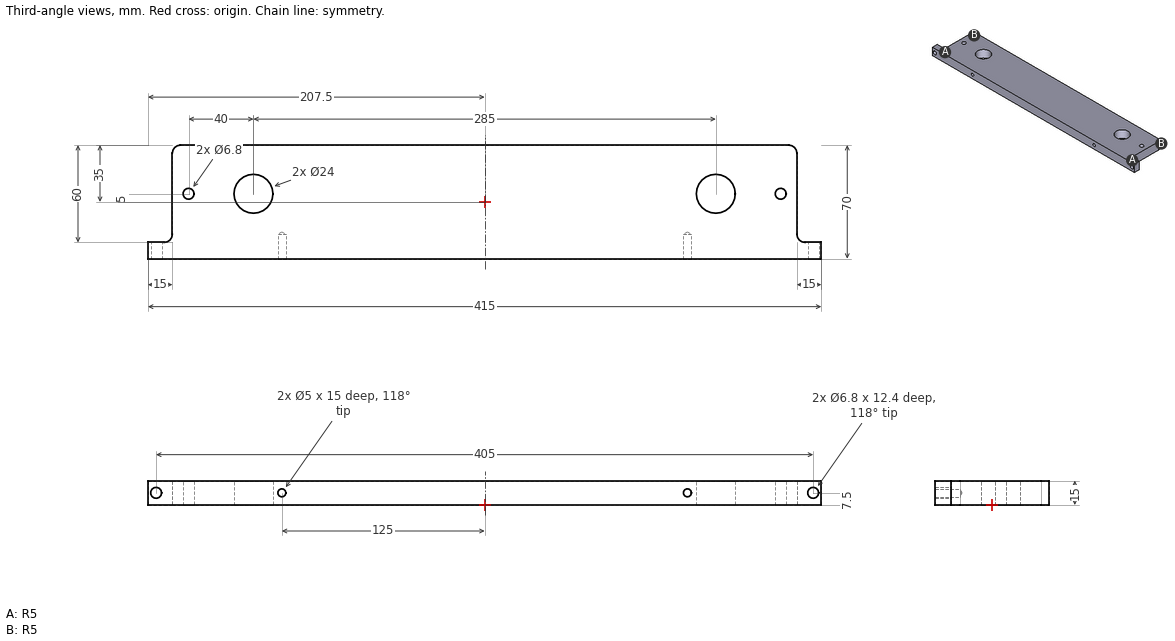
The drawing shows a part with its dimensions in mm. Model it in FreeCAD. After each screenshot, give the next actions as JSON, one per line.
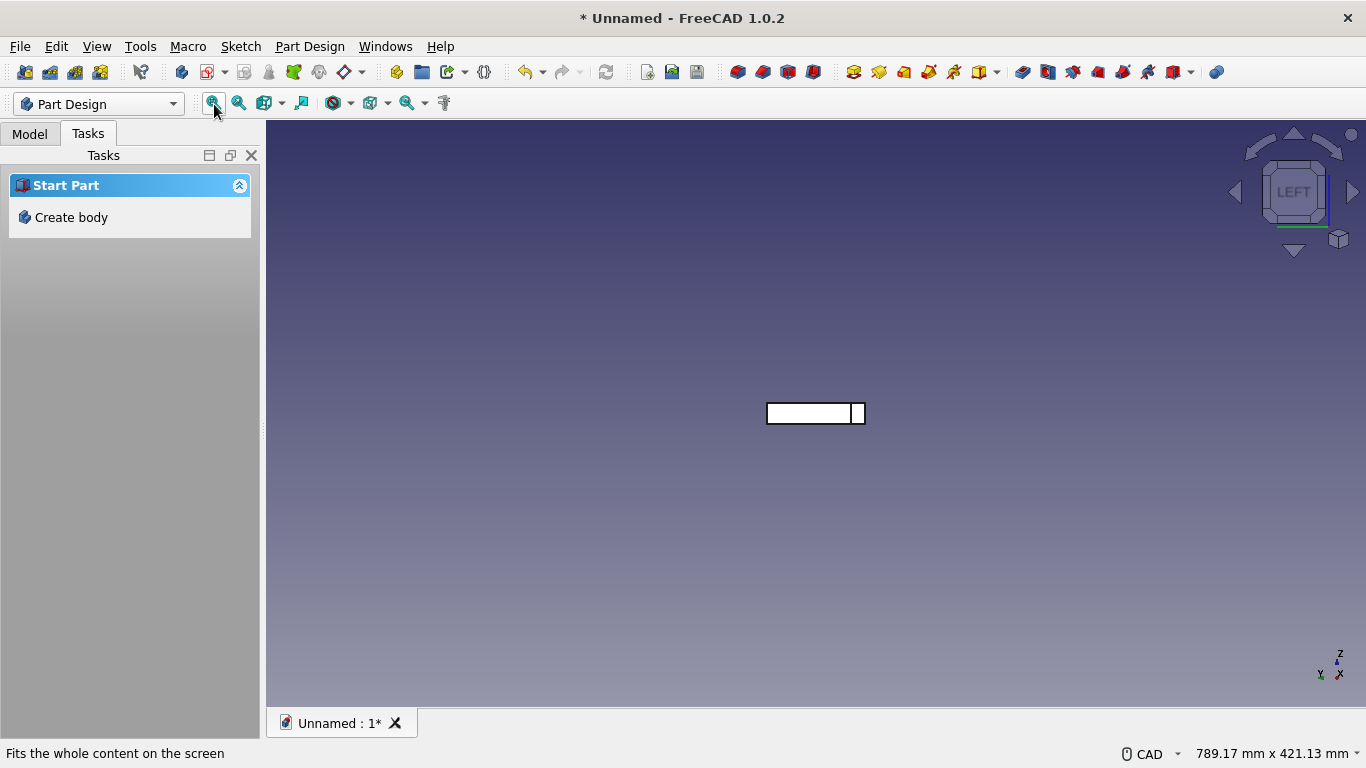
{"action": "scroll", "coordinate": [851, 412], "scroll_direction": "up", "scroll_amount": 4}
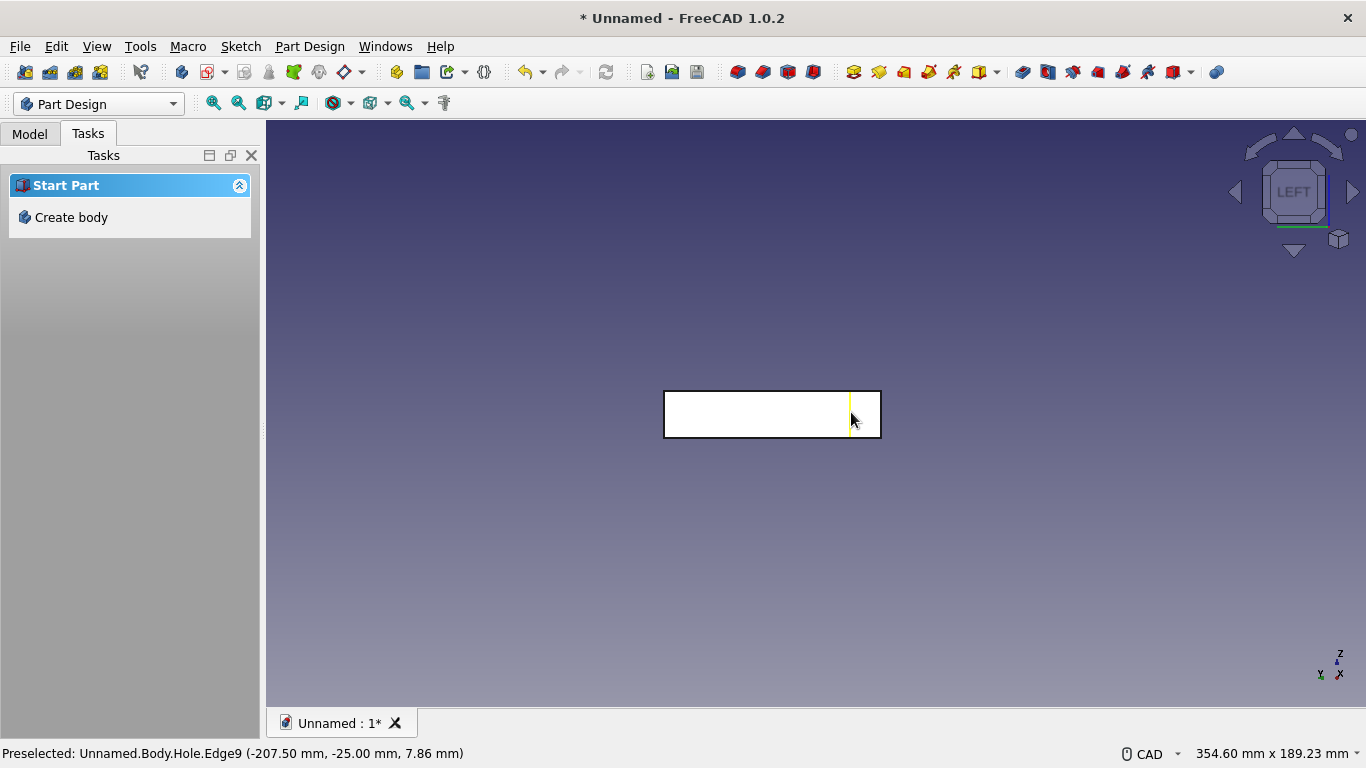
{"action": "key", "text": "v f"}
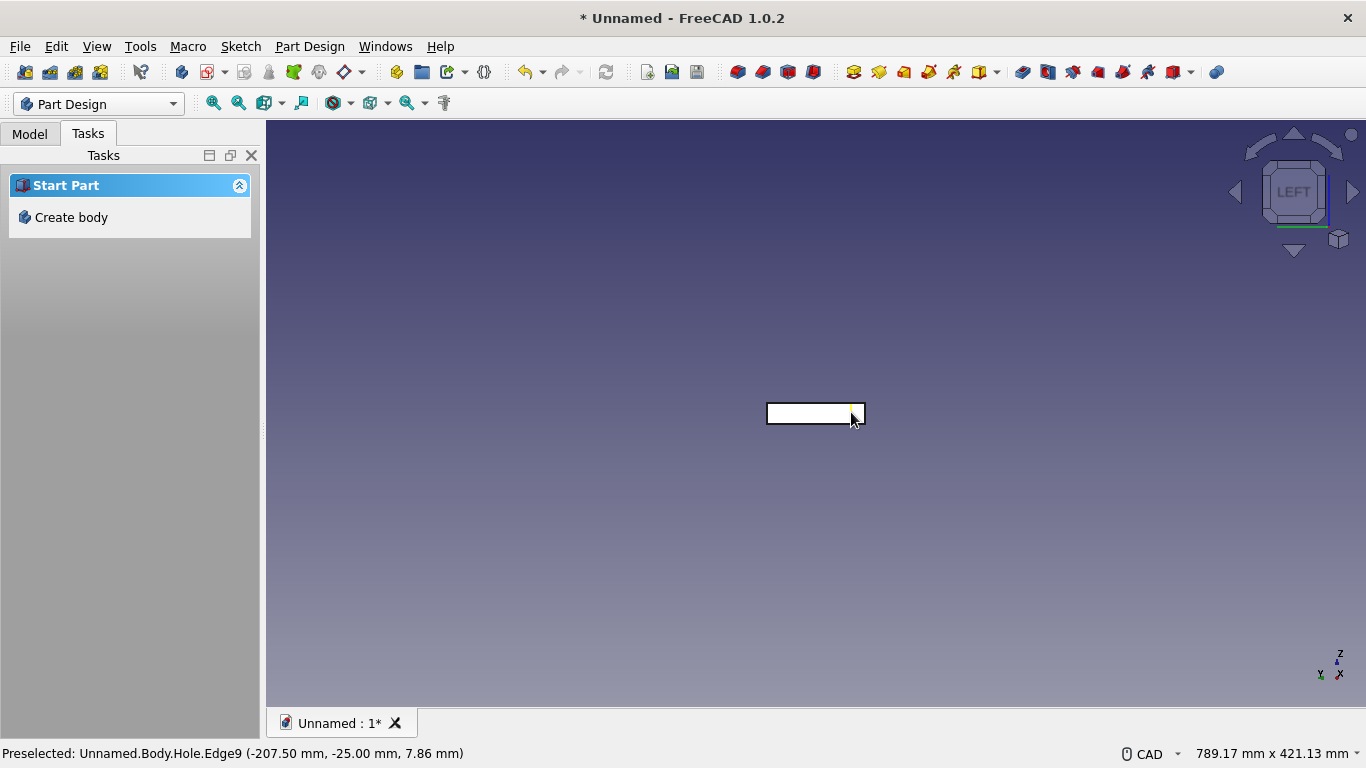
{"action": "key", "text": "v 3"}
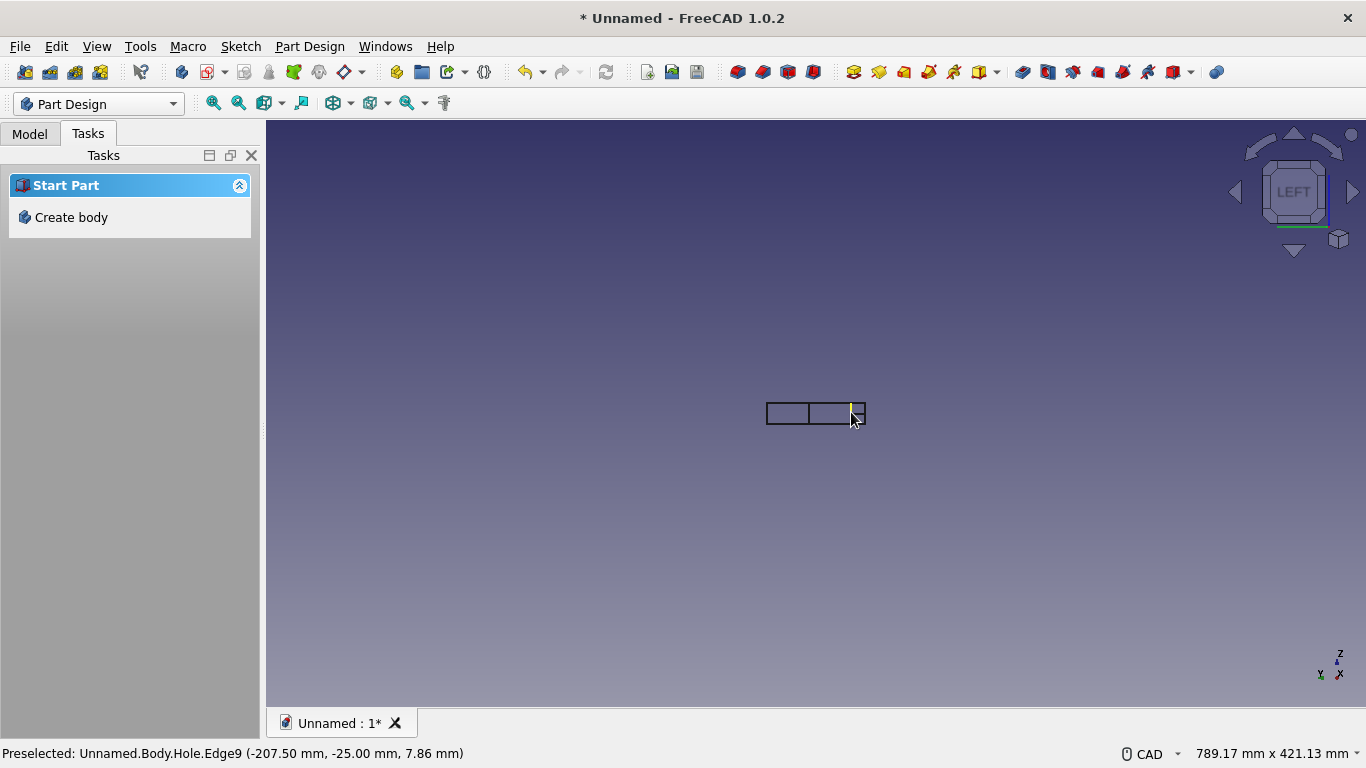
{"action": "key", "text": "0"}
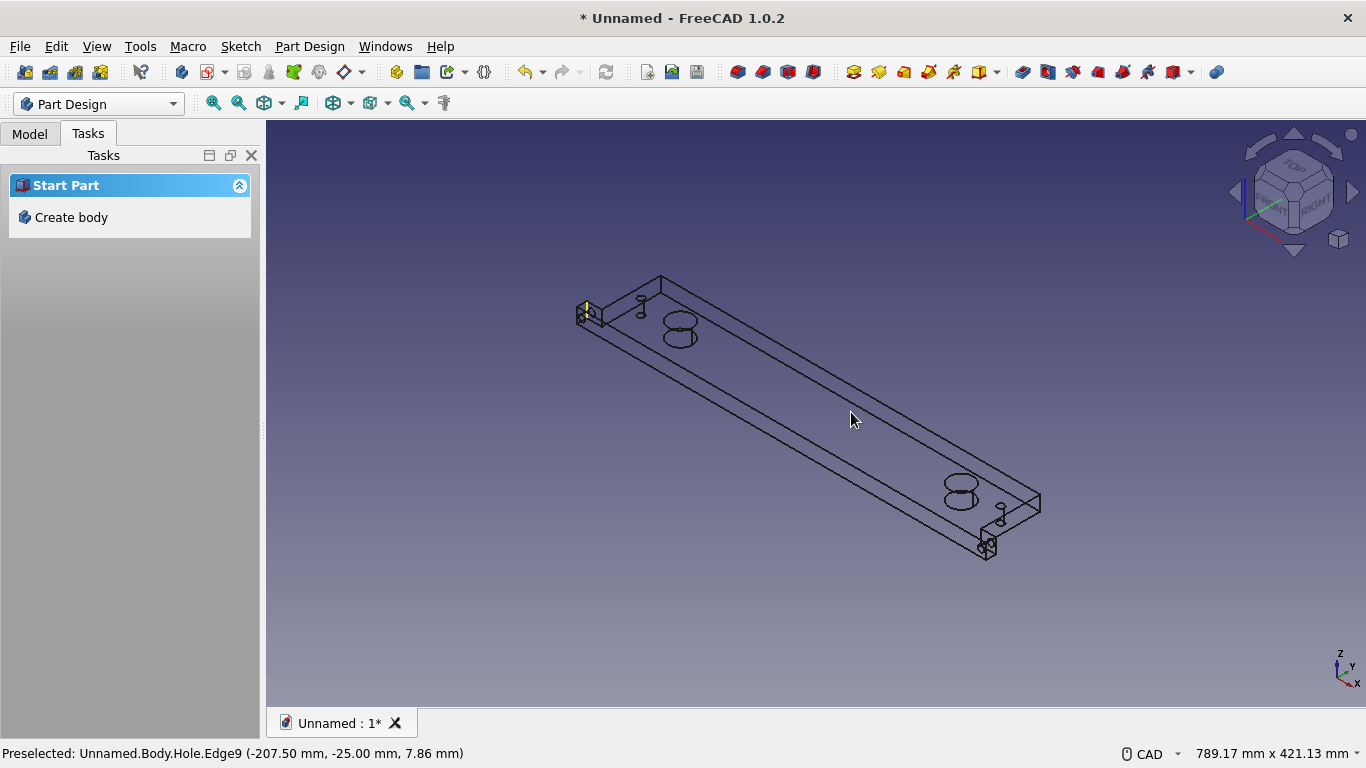
{"action": "scroll", "coordinate": [602, 317], "scroll_direction": "up", "scroll_amount": 6}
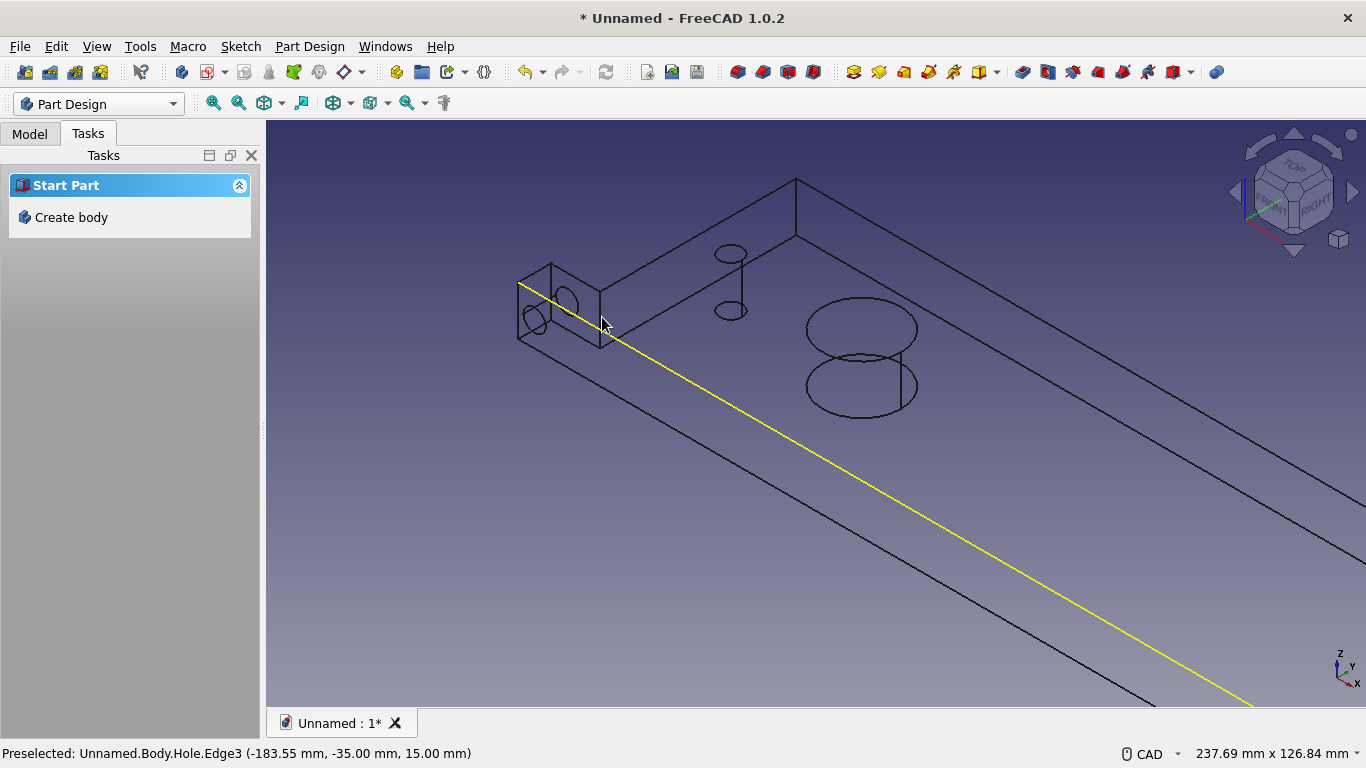
{"action": "left_click", "coordinate": [600, 319]}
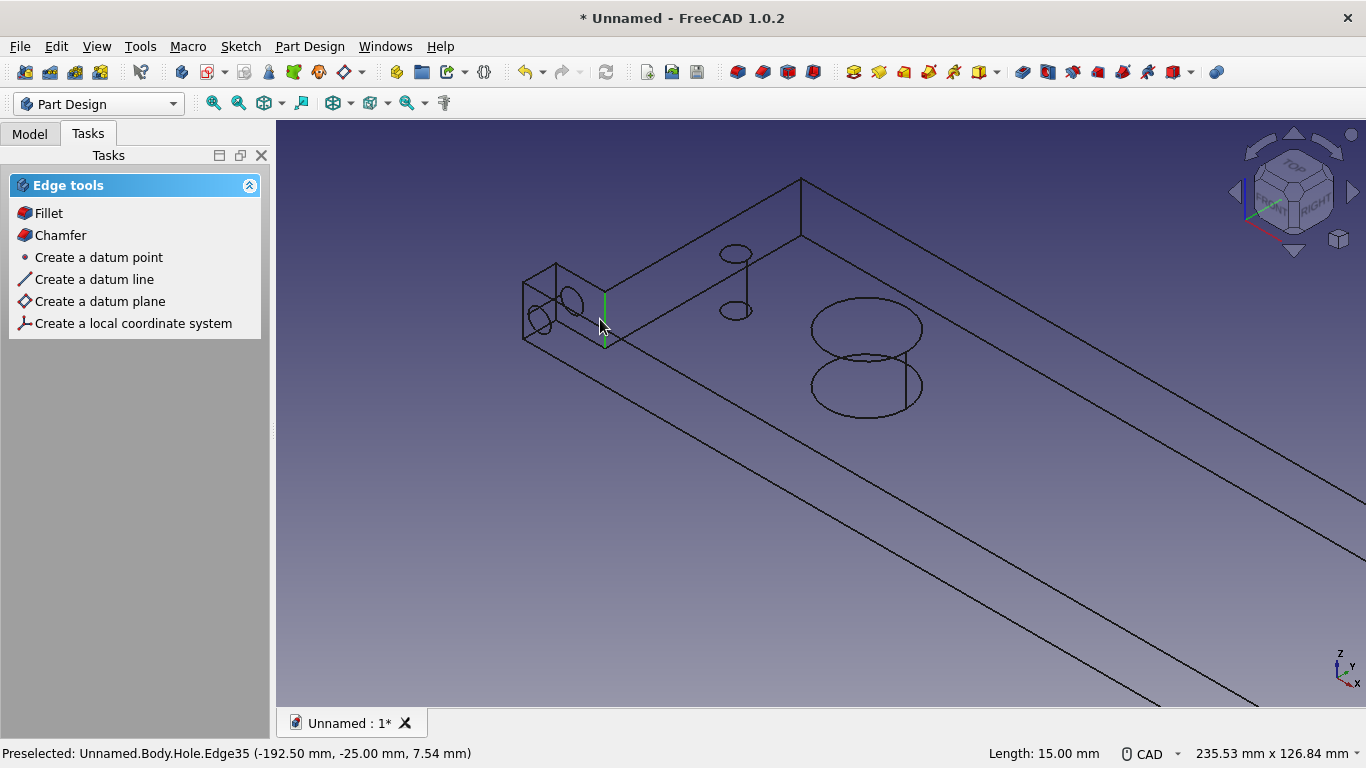
{"action": "key", "text": "v f"}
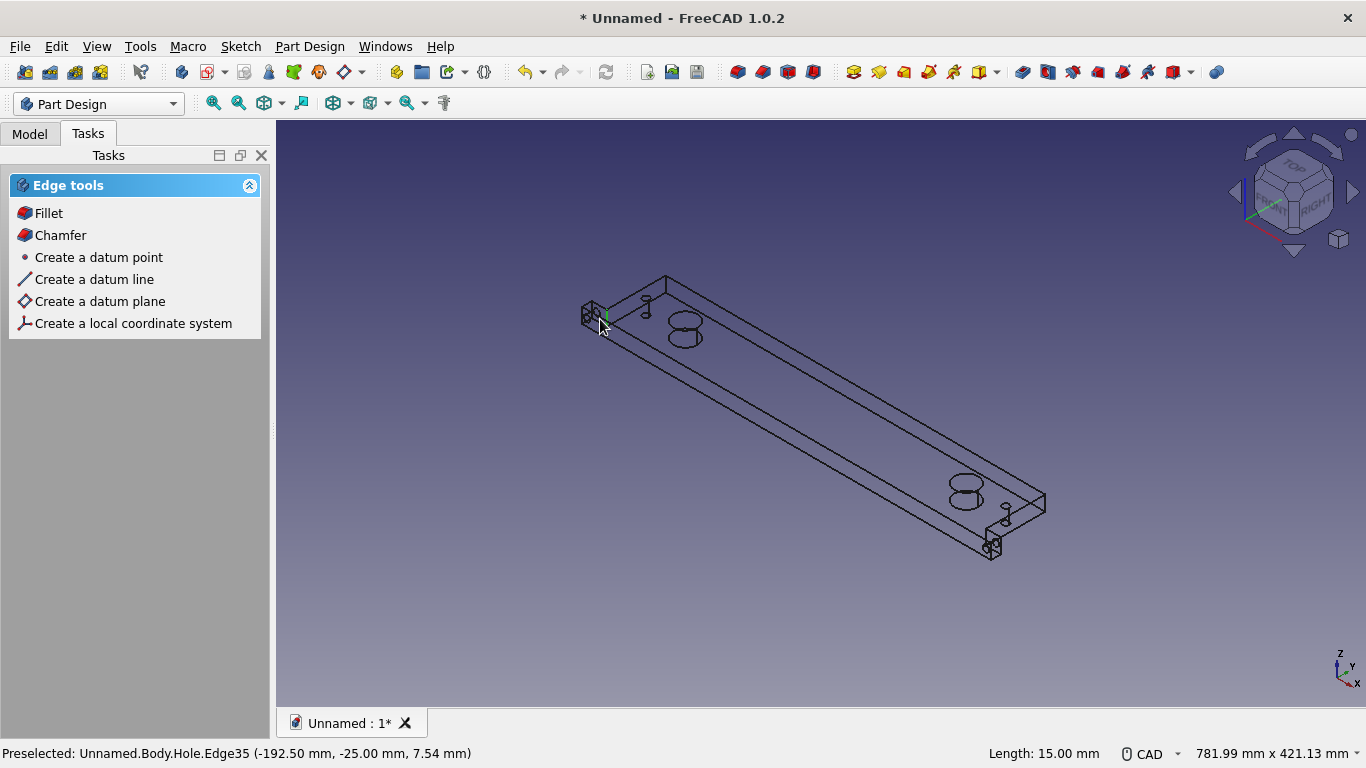
{"action": "key", "text": "2"}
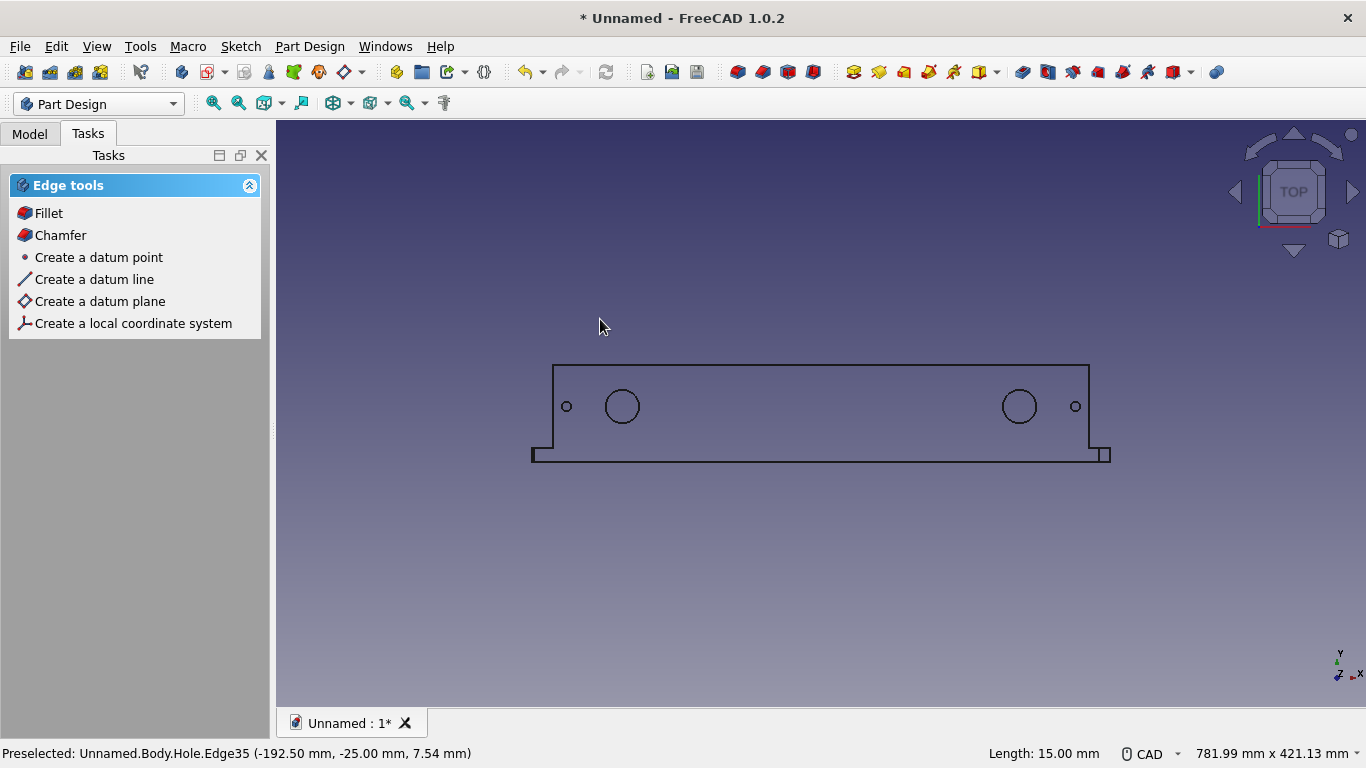
{"action": "scroll", "coordinate": [1089, 447], "scroll_direction": "up", "scroll_amount": 6}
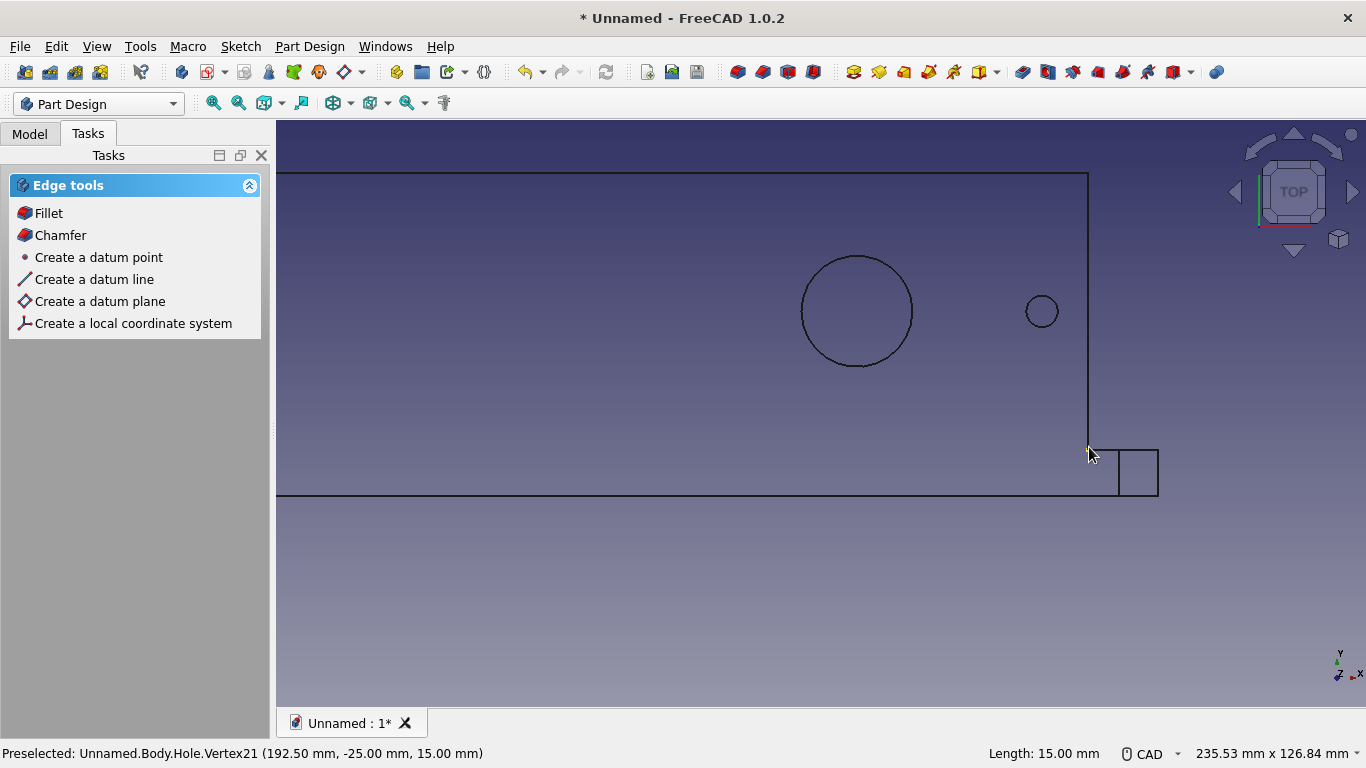
{"action": "key", "text": "v f"}